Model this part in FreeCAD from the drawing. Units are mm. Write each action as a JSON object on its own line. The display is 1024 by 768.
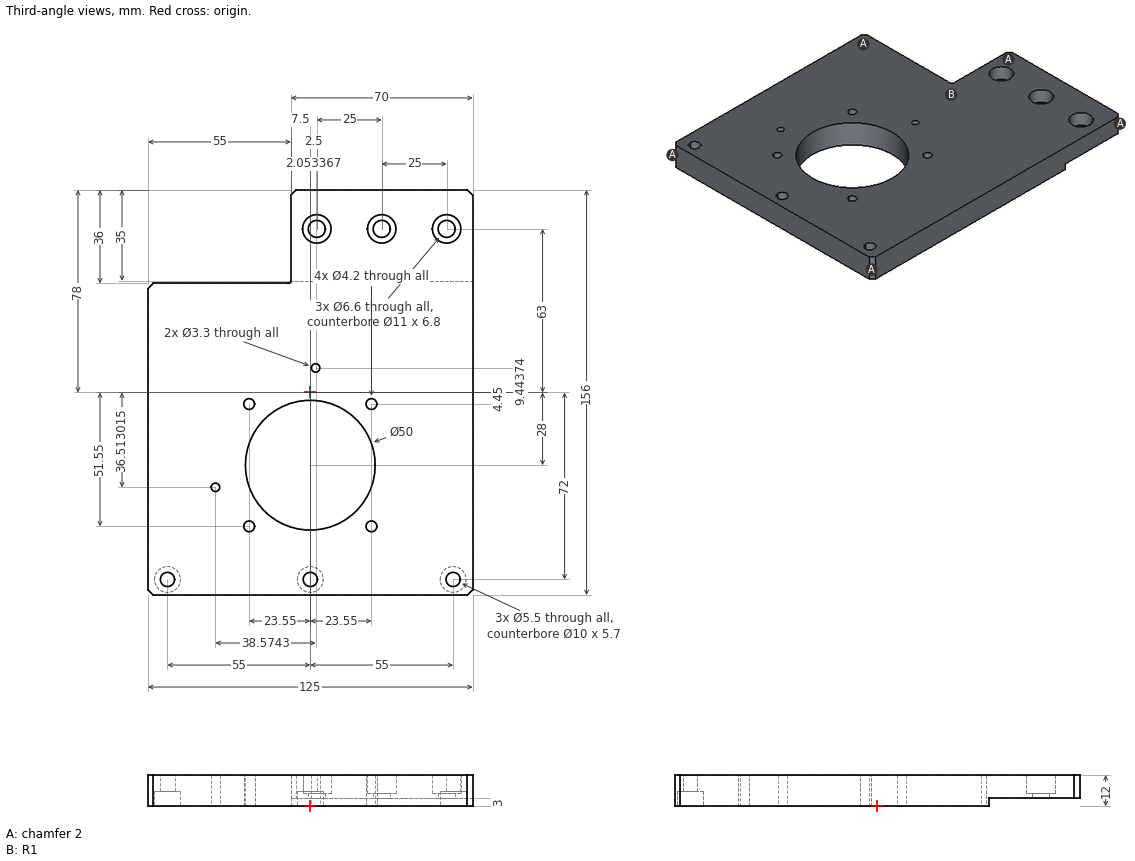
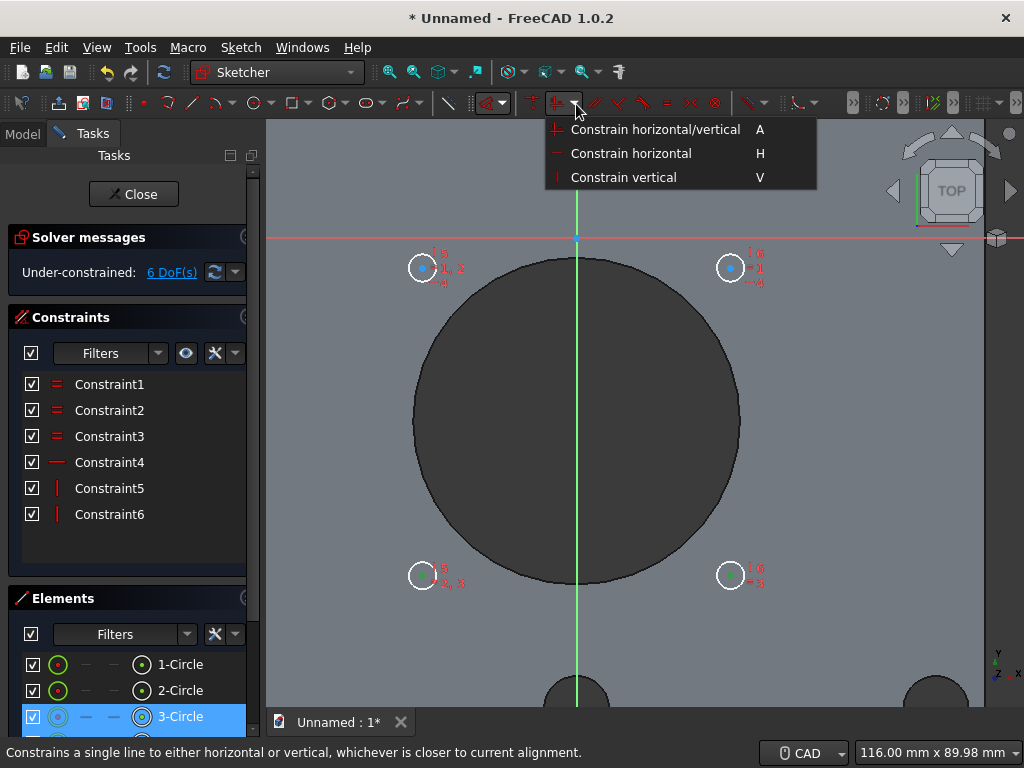
{"action": "left_click", "coordinate": [681, 153]}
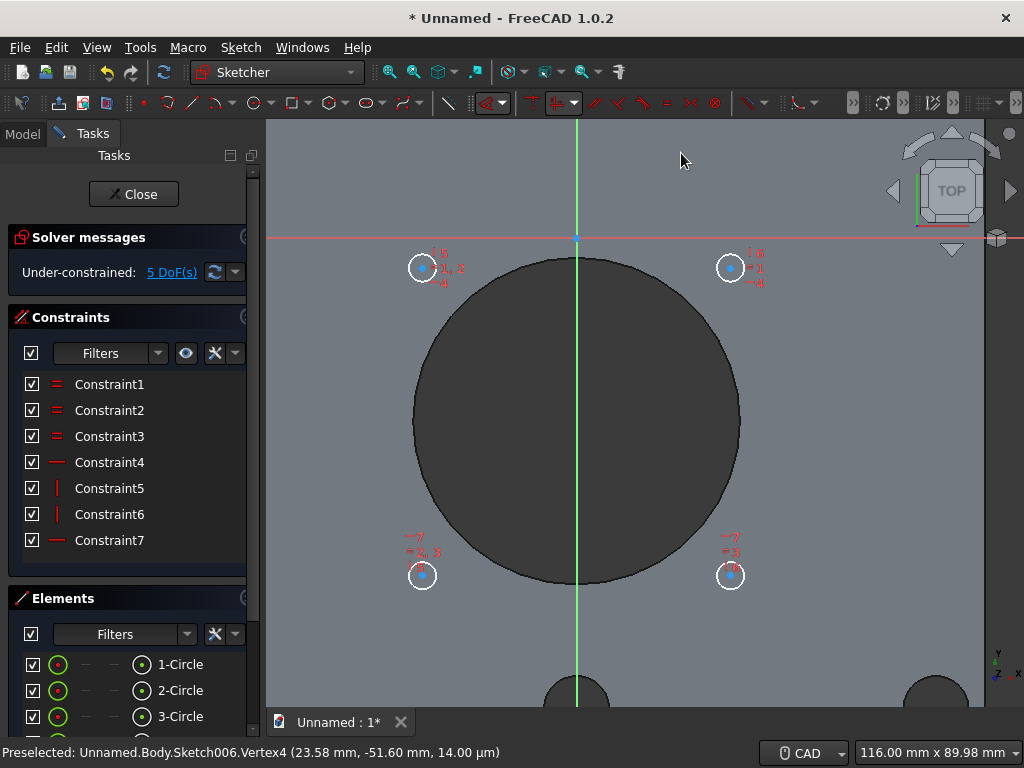
{"action": "scroll", "coordinate": [740, 258], "scroll_direction": "up", "scroll_amount": 2}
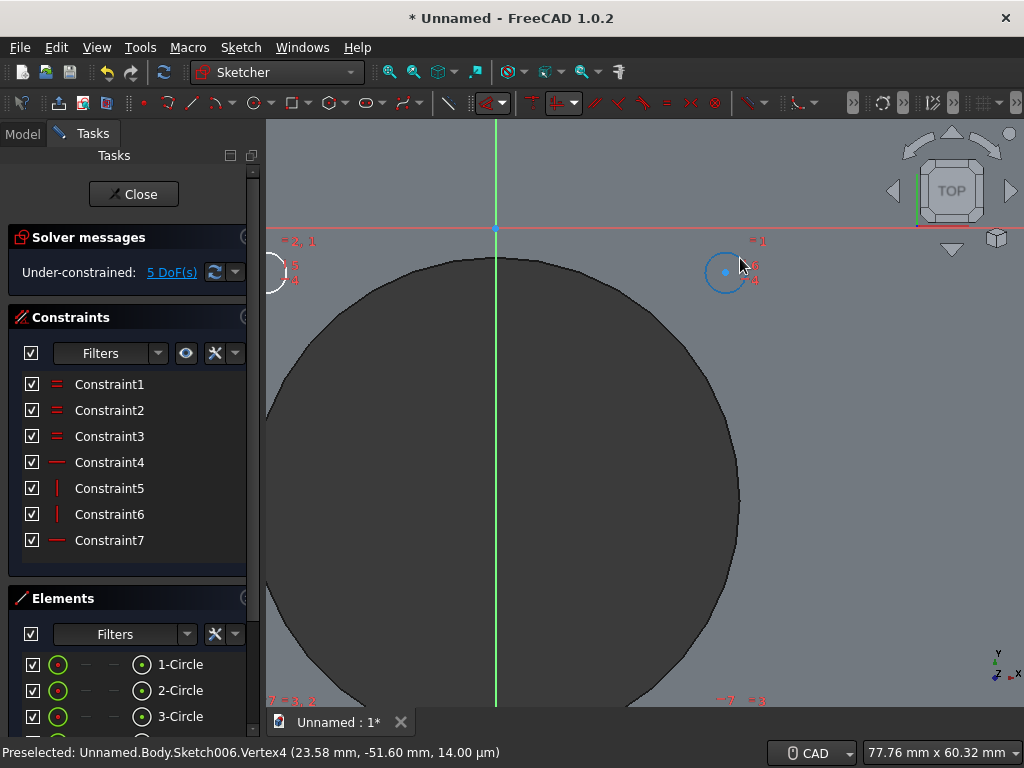
{"action": "left_click", "coordinate": [711, 259]}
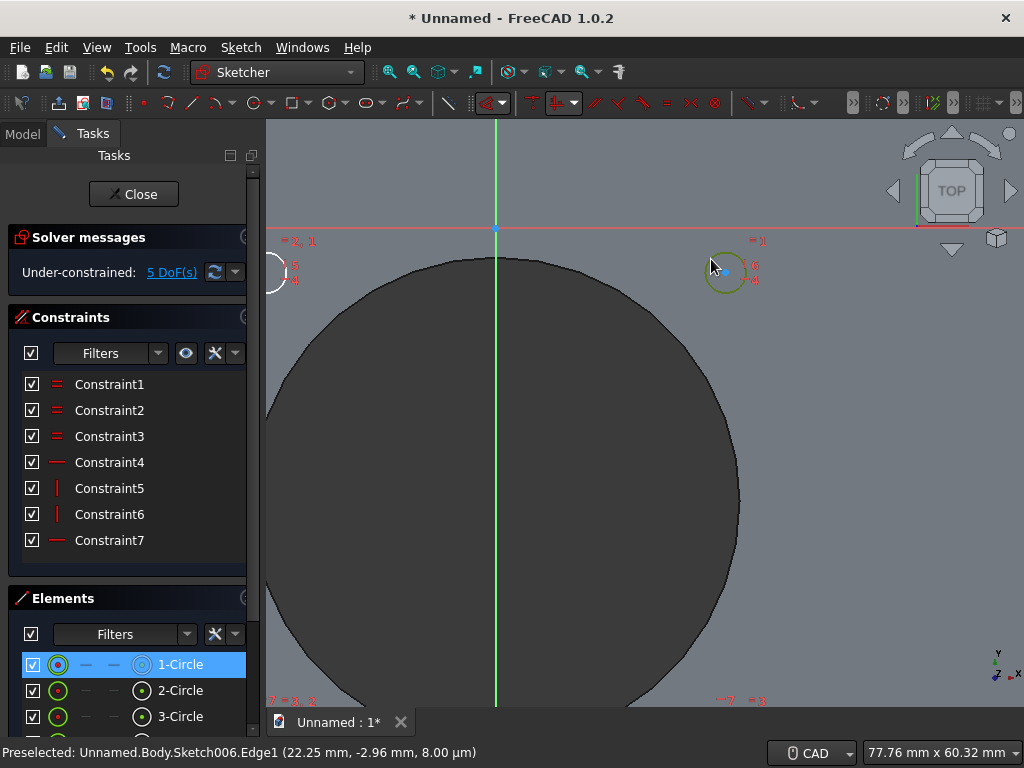
{"action": "key", "text": "k o"}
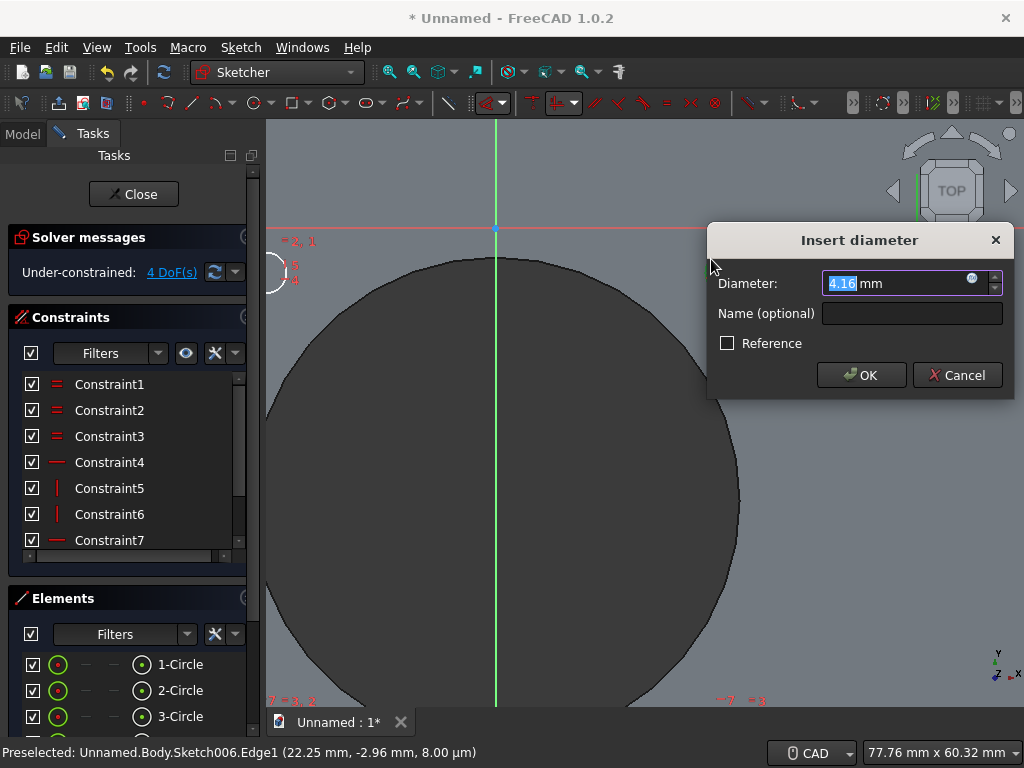
{"action": "type", "text": "4.2"}
{"action": "key", "text": "Return"}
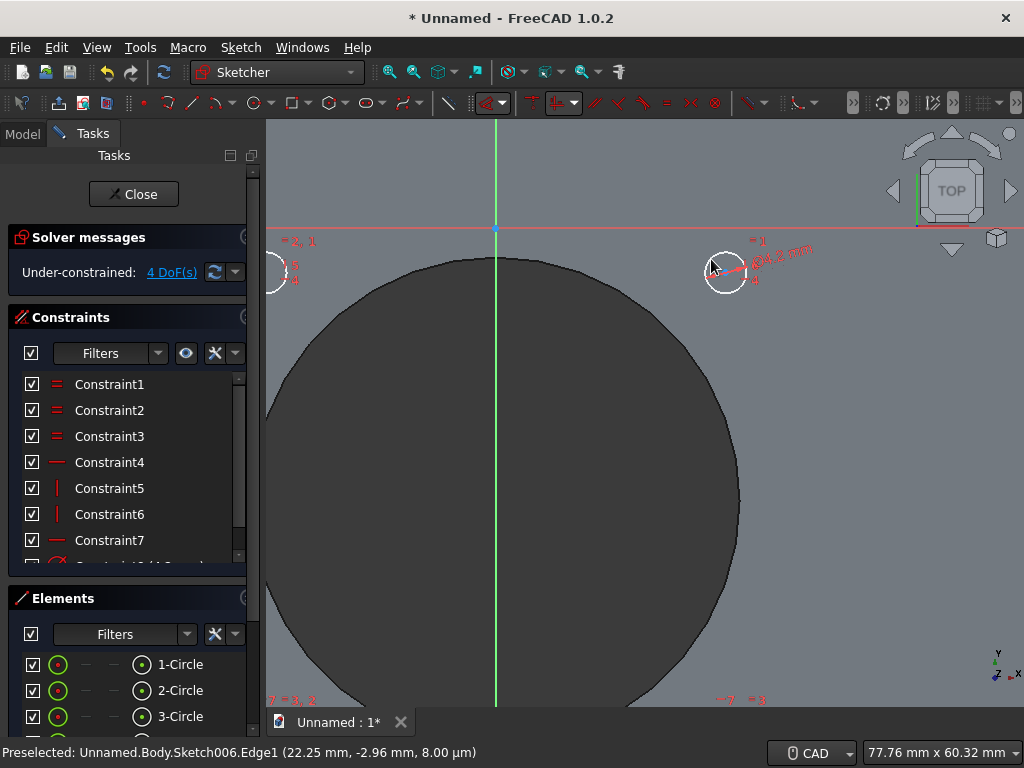
{"action": "left_click", "coordinate": [726, 273]}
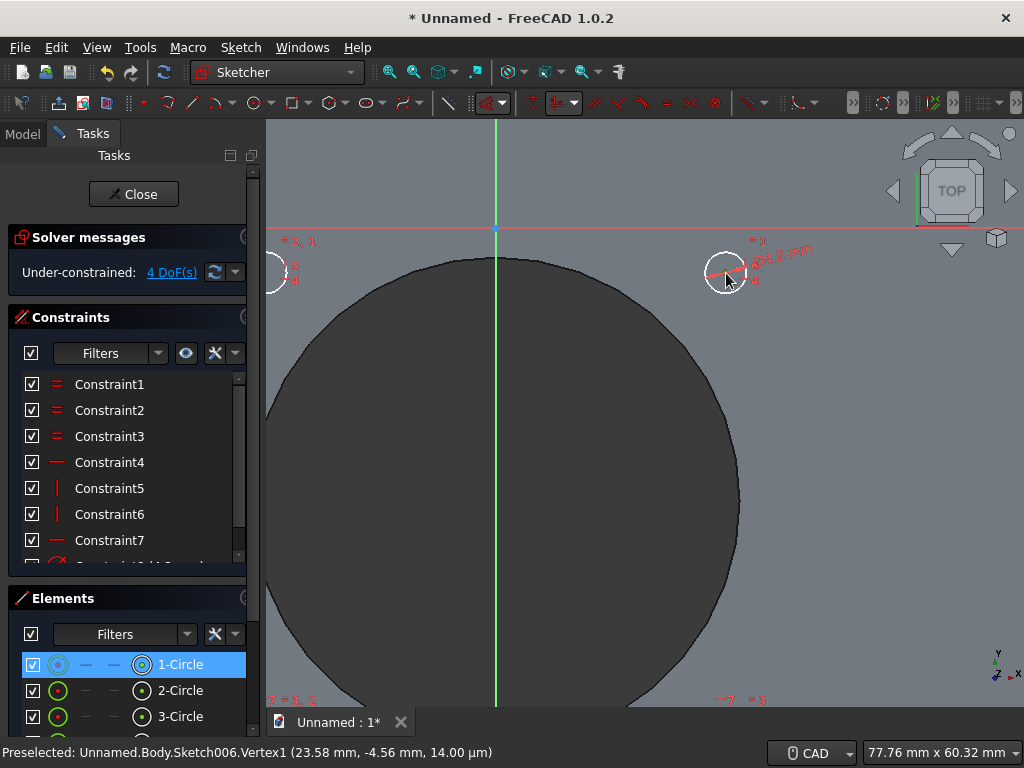
{"action": "key", "text": "i"}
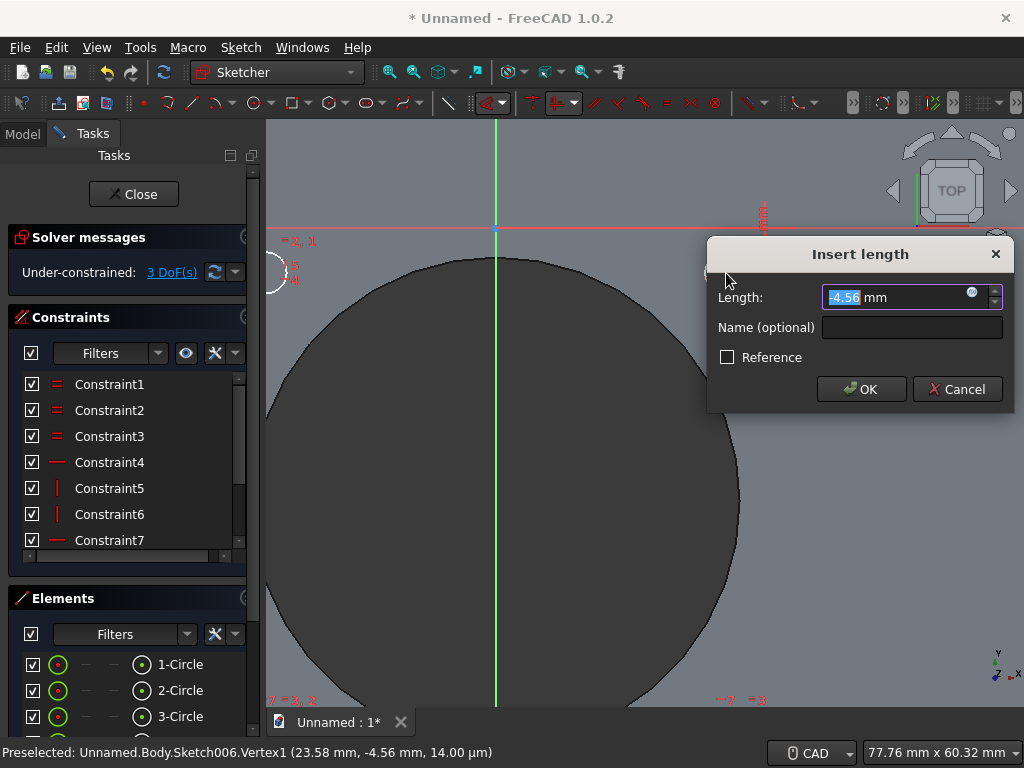
{"action": "type", "text": "-4.45"}
{"action": "key", "text": "Return"}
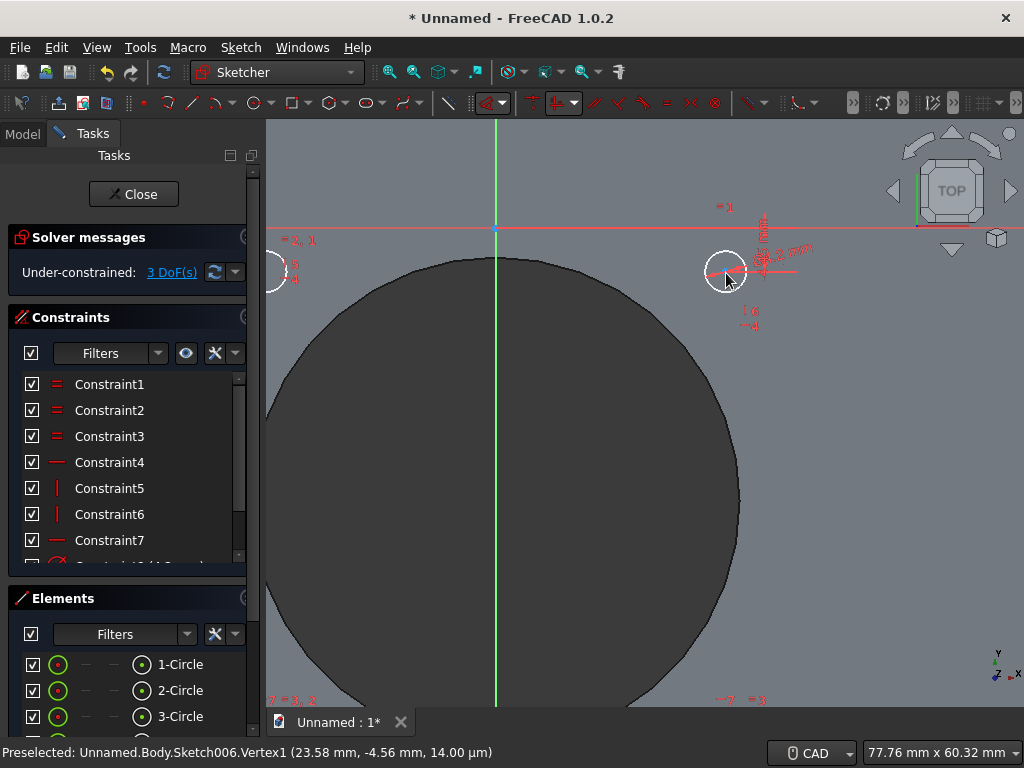
{"action": "left_click", "coordinate": [726, 272]}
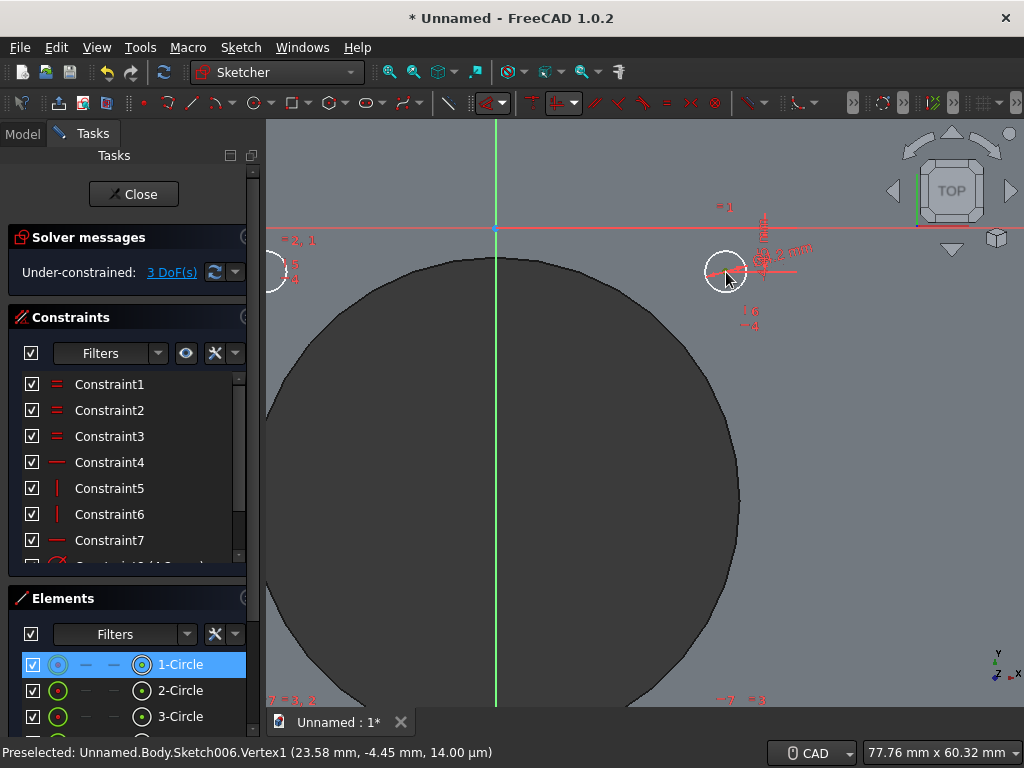
{"action": "left_click", "coordinate": [504, 104]}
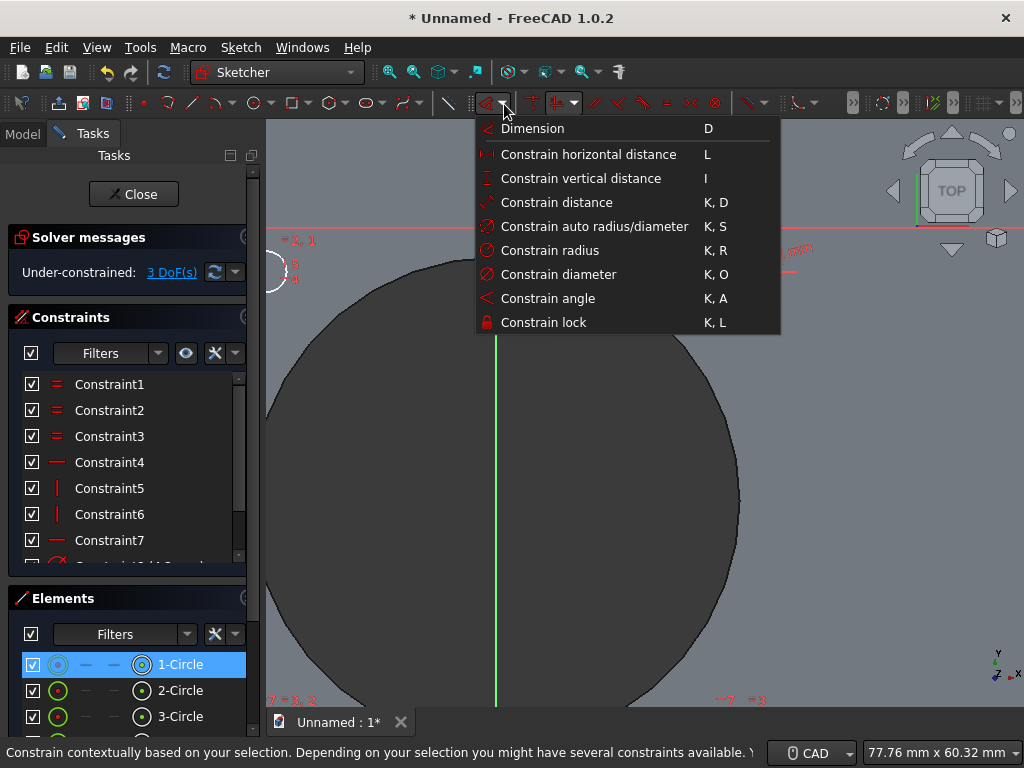
{"action": "left_click", "coordinate": [628, 154]}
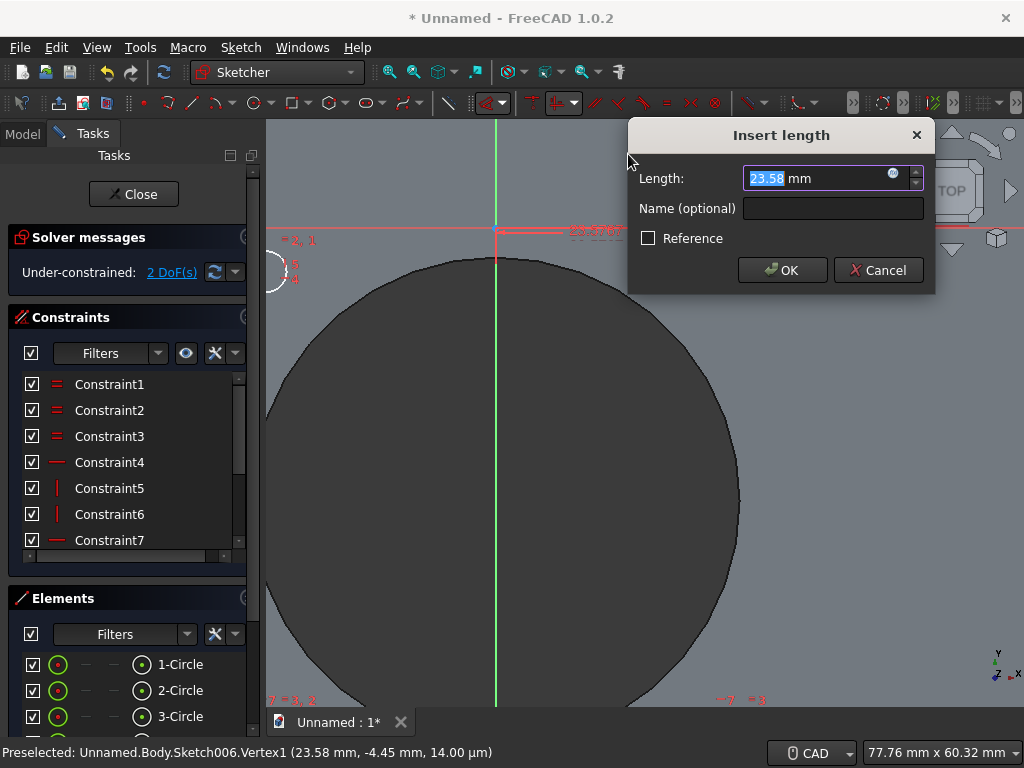
{"action": "type", "text": "23.55"}
{"action": "key", "text": "Return"}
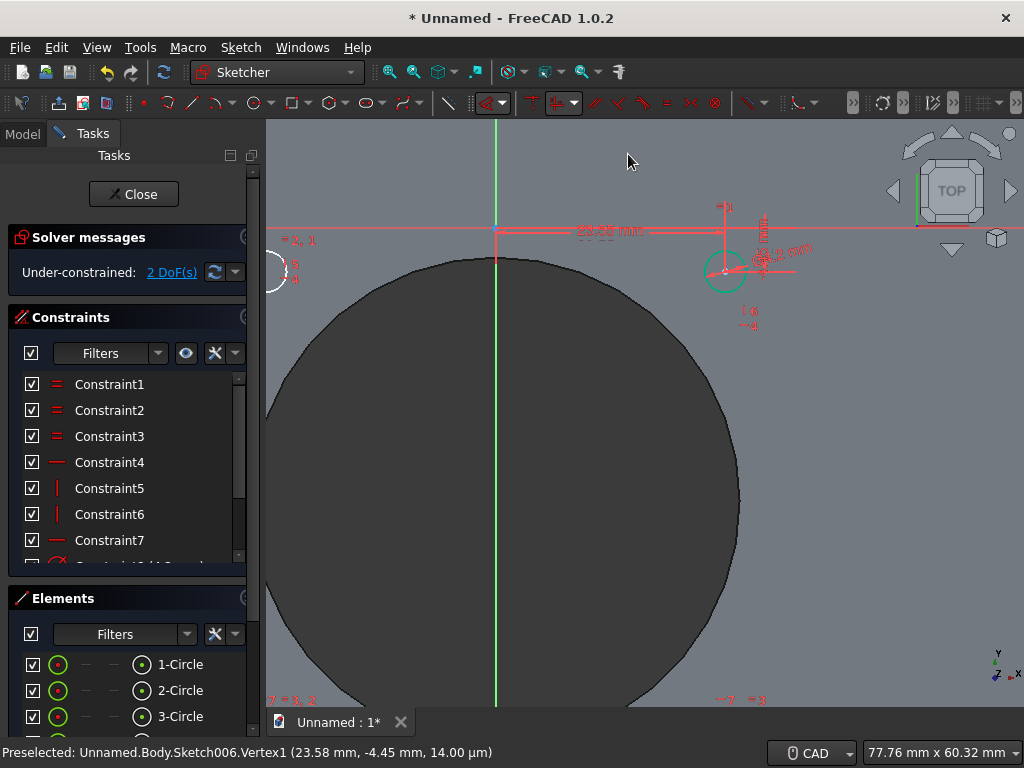
{"action": "scroll", "coordinate": [740, 257], "scroll_direction": "down", "scroll_amount": 2}